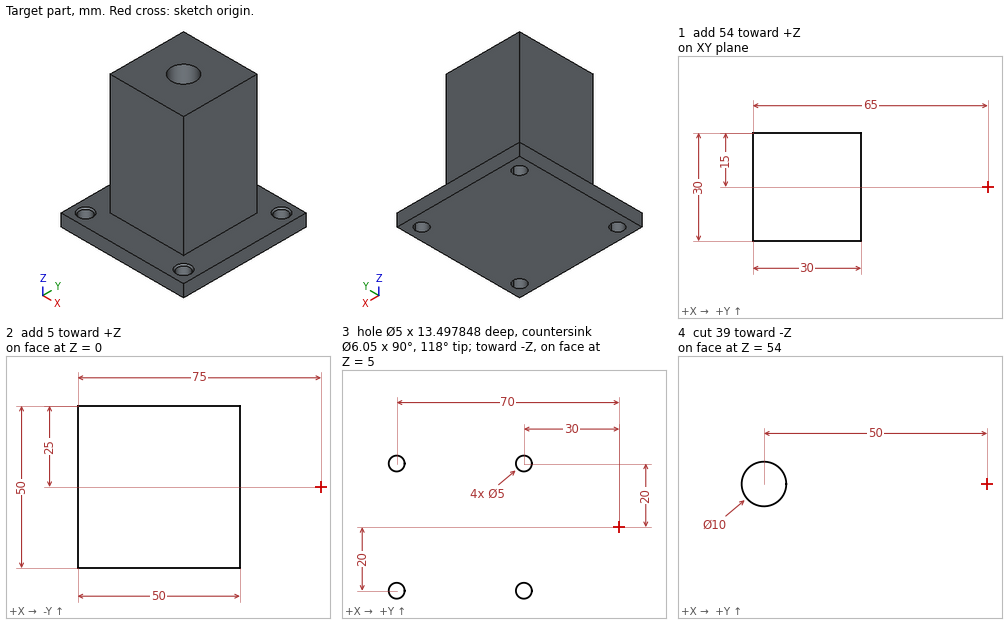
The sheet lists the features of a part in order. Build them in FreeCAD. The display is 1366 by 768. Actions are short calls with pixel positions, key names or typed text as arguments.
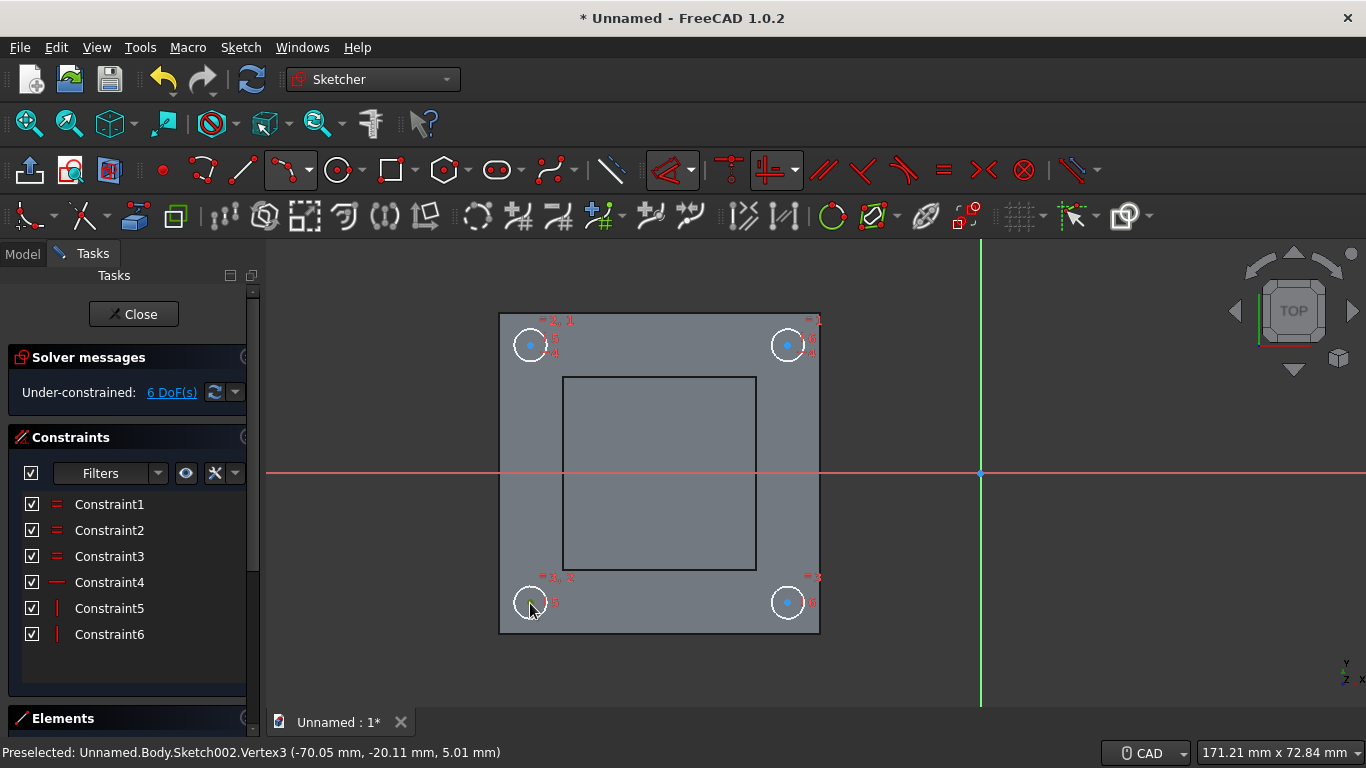
click(788, 603)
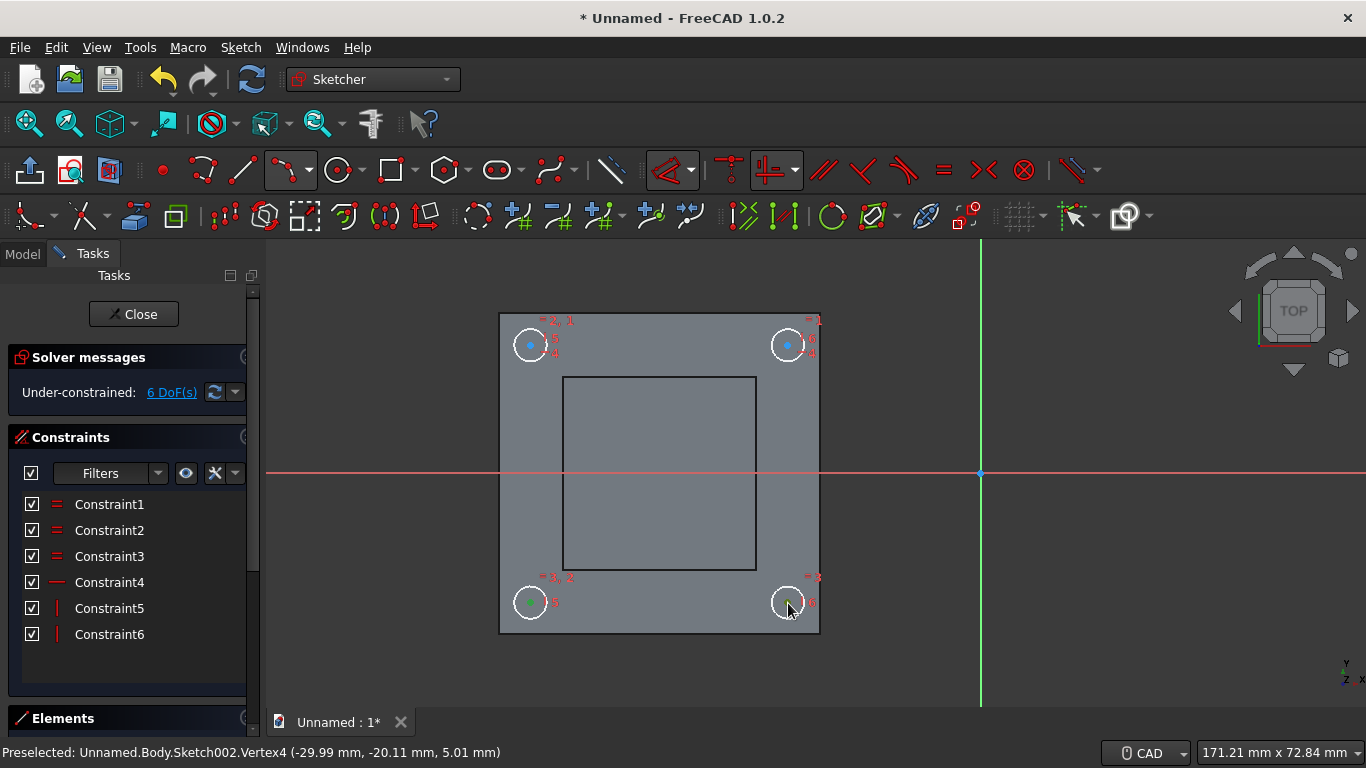
key(h)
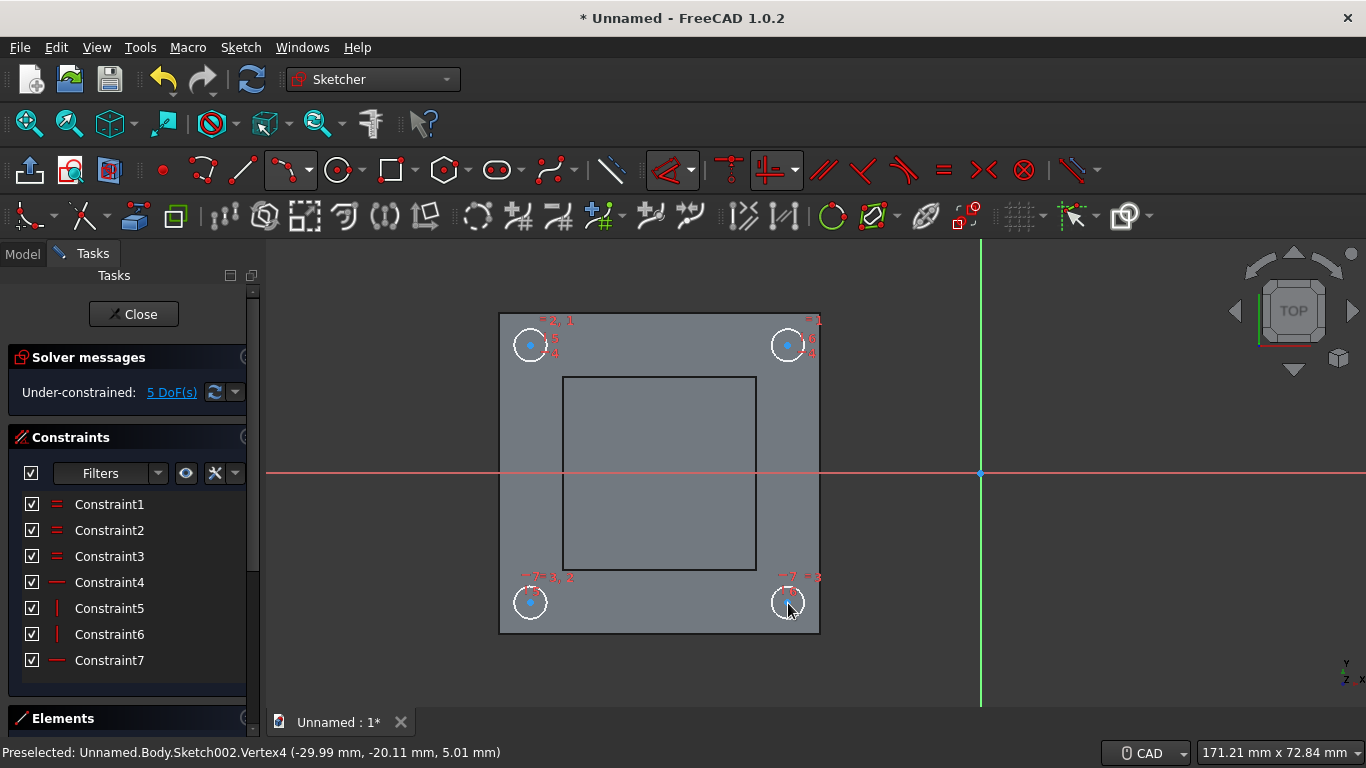
key(d)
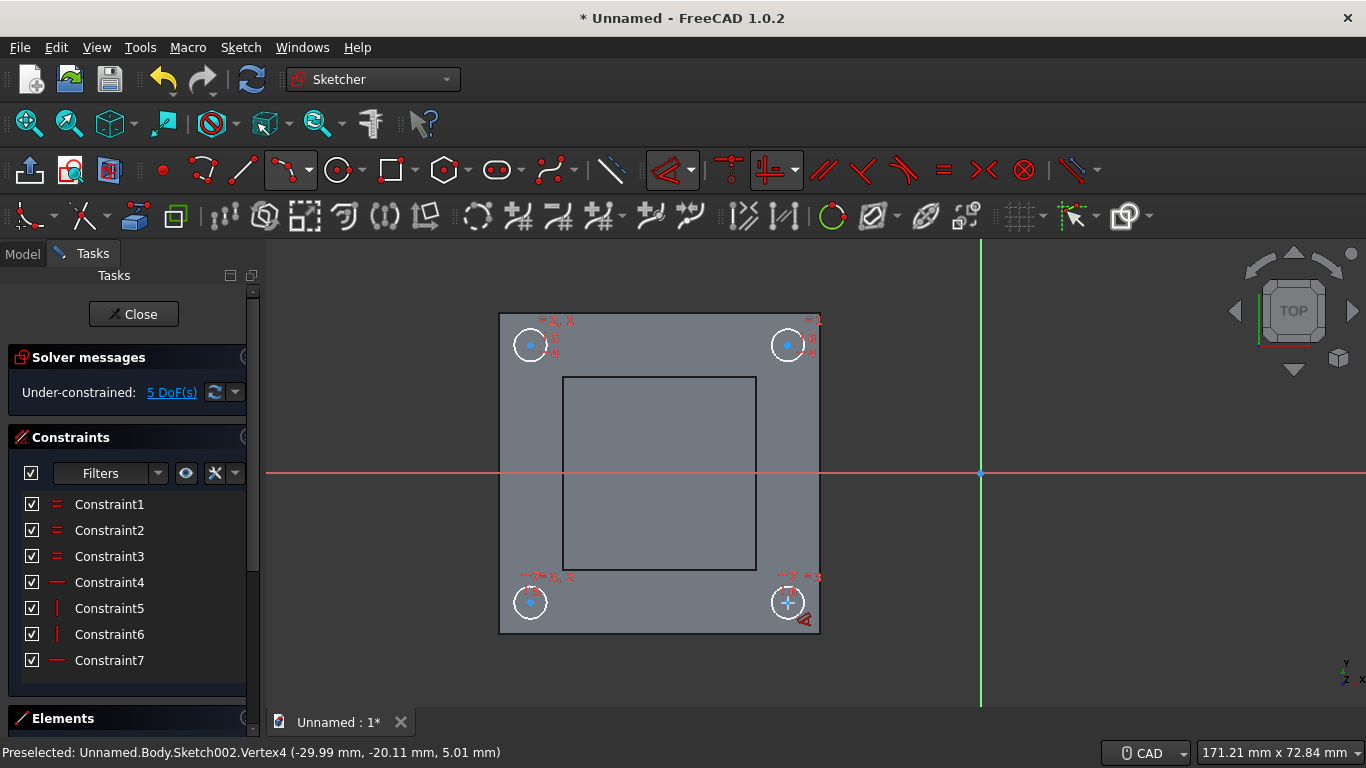
scroll(799, 334, up, 2)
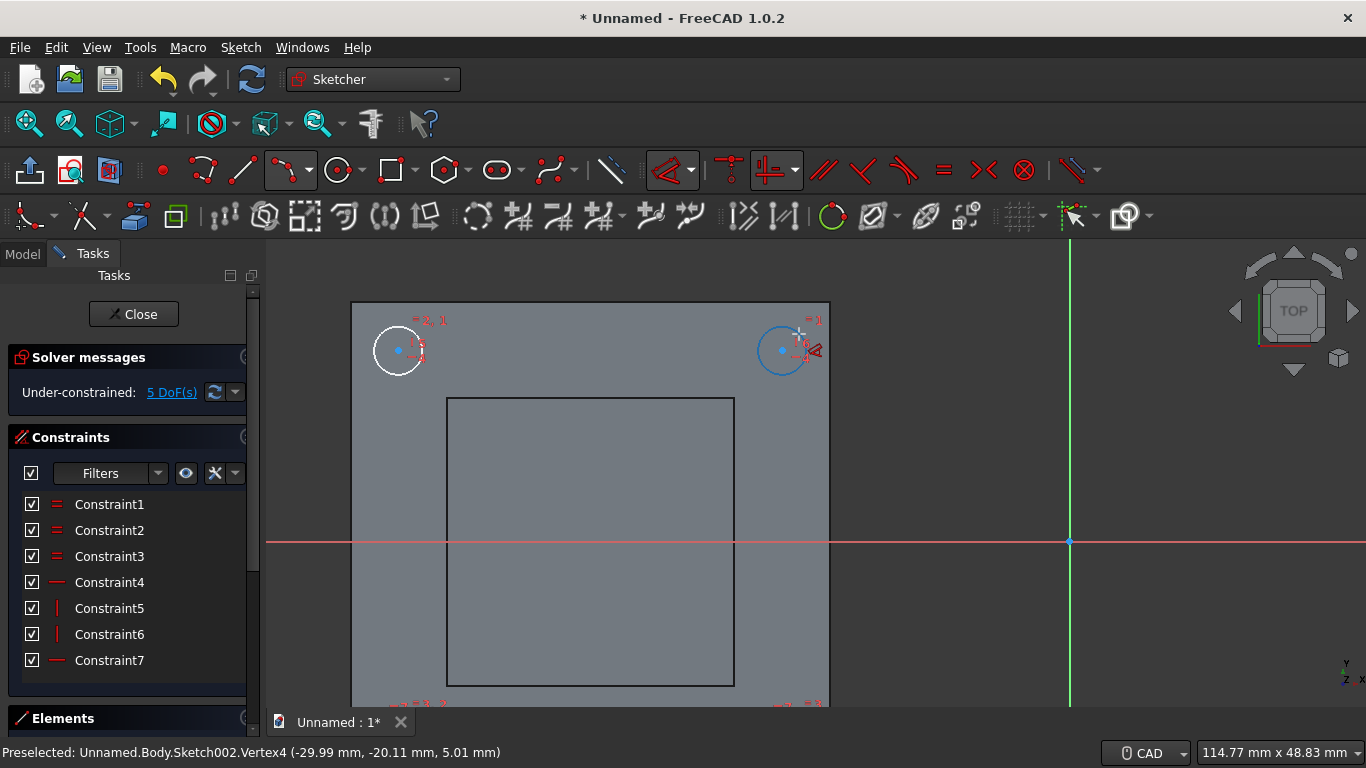
click(799, 334)
click(822, 311)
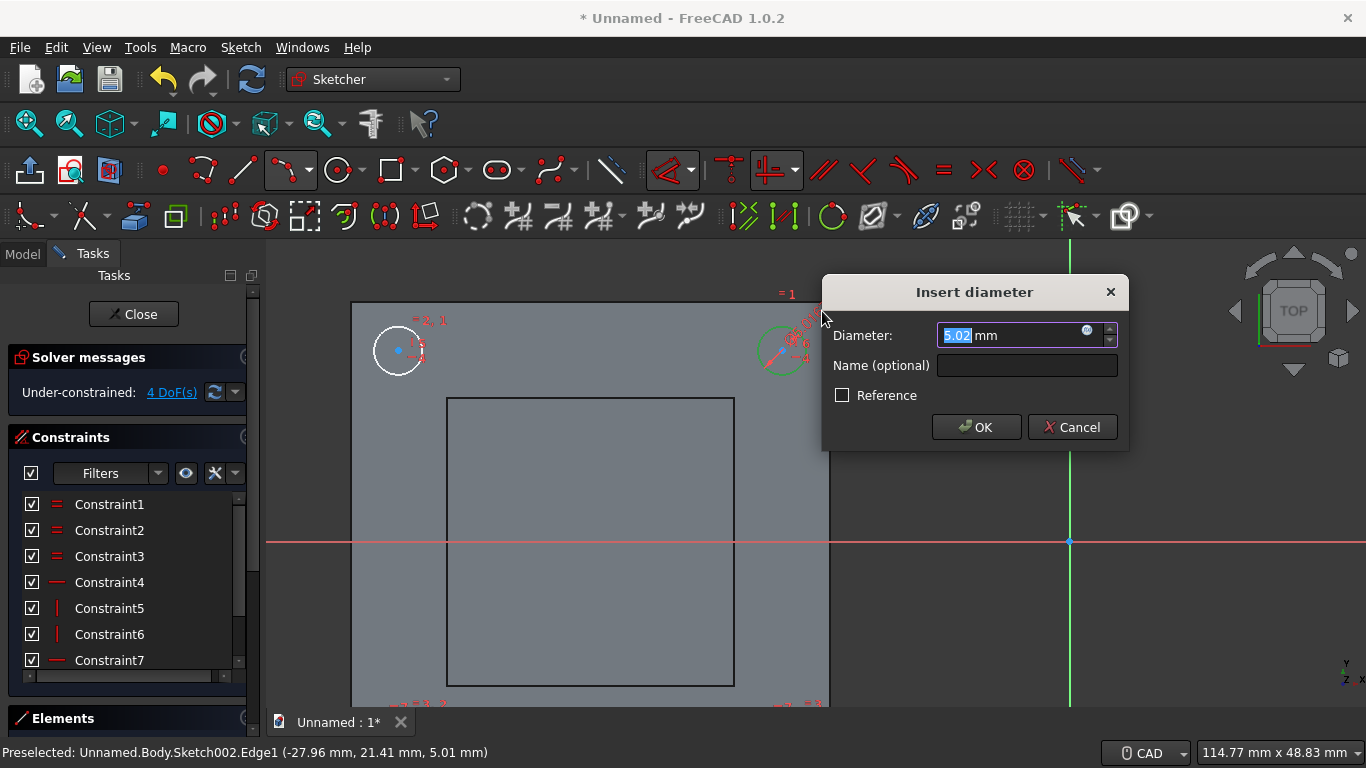
text(5)
key(Return)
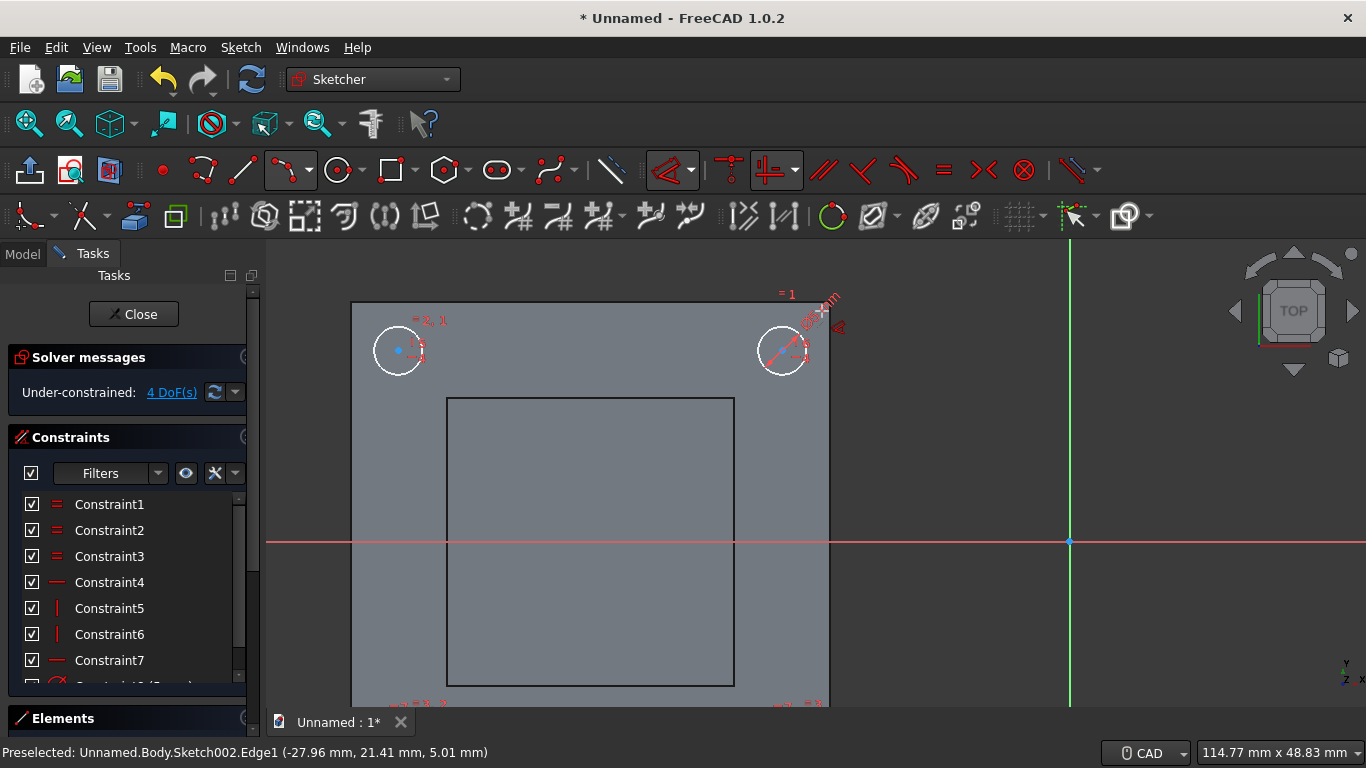
click(782, 351)
click(926, 317)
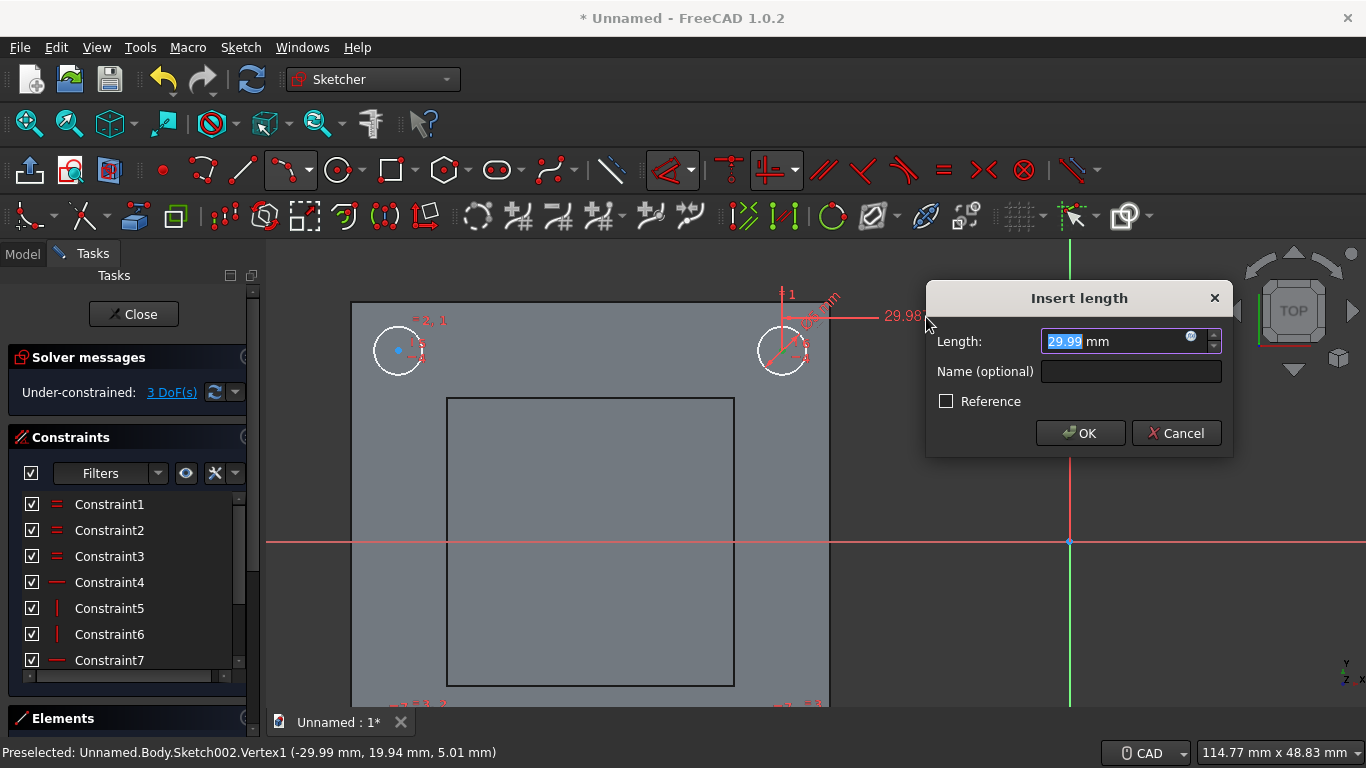
text(30)
key(Return)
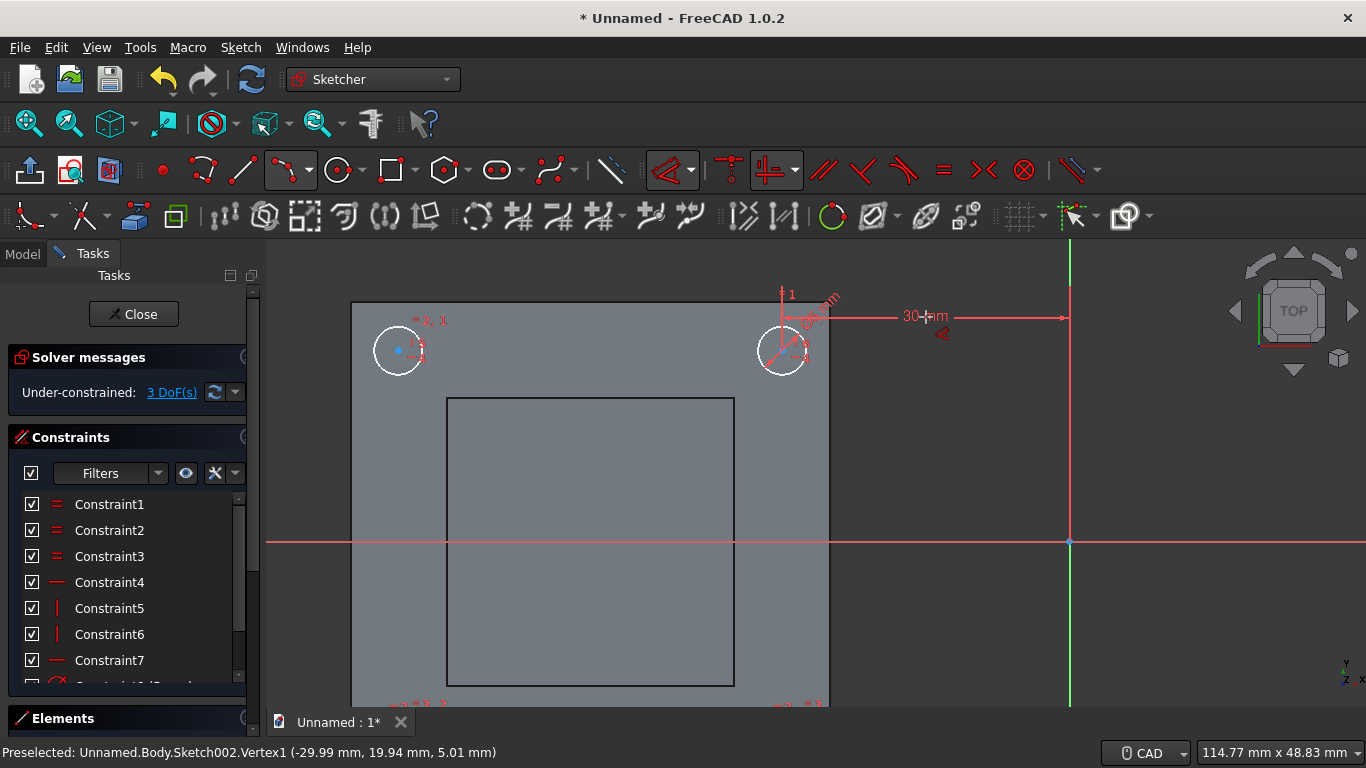
click(782, 351)
click(1104, 446)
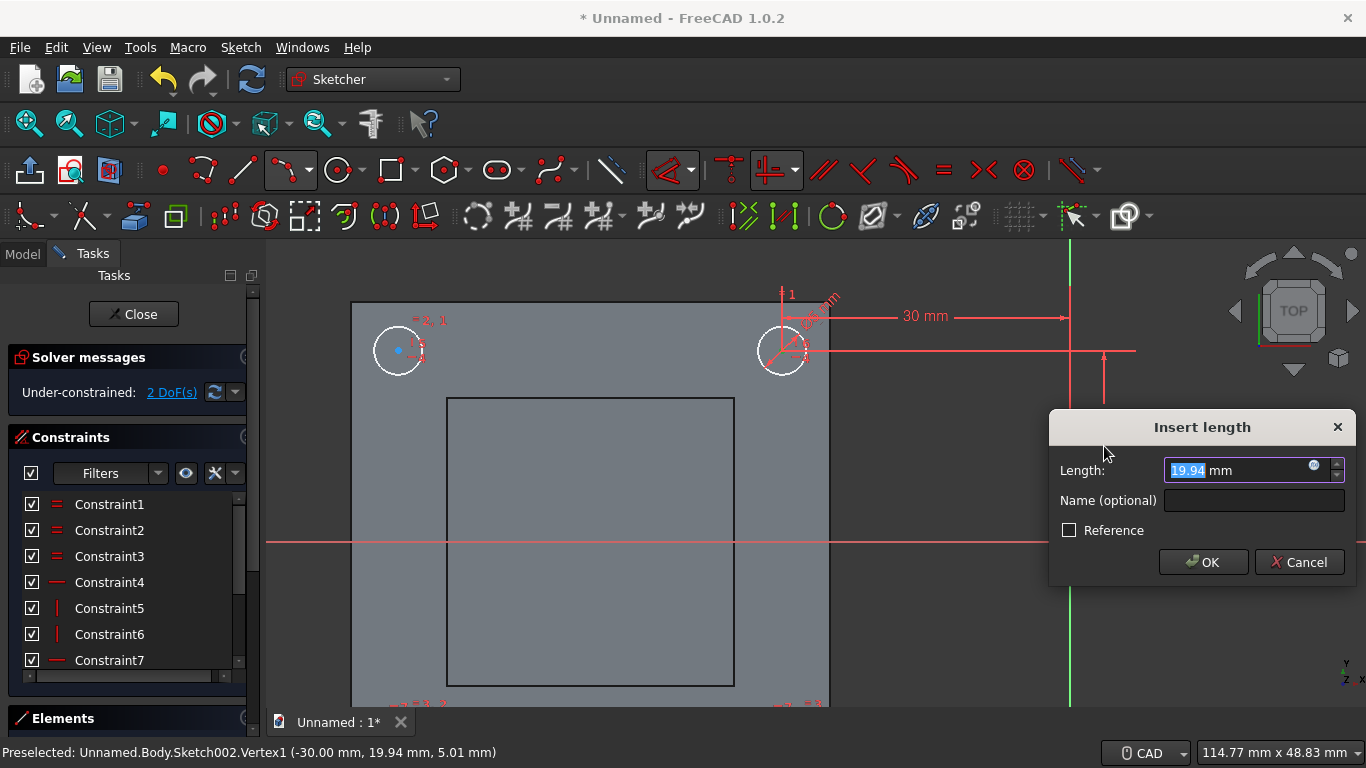
text(20)
key(Return)